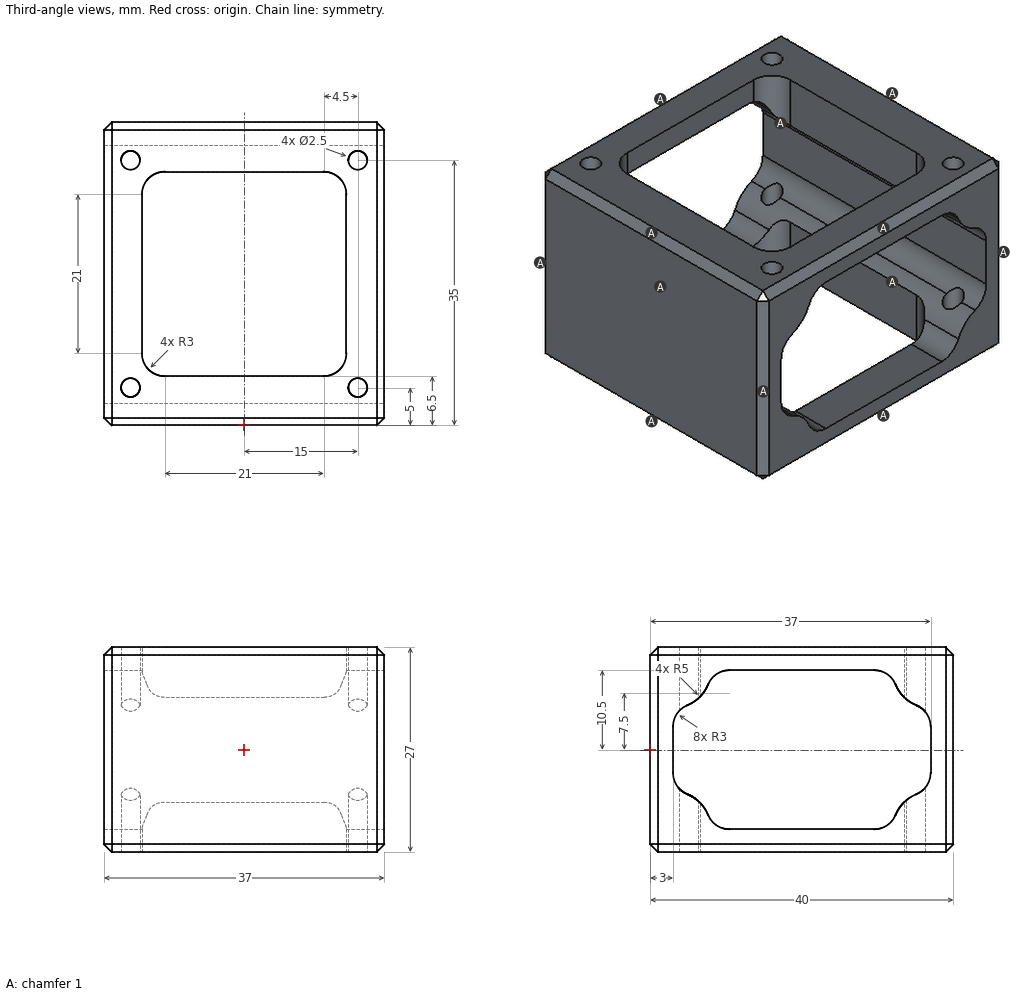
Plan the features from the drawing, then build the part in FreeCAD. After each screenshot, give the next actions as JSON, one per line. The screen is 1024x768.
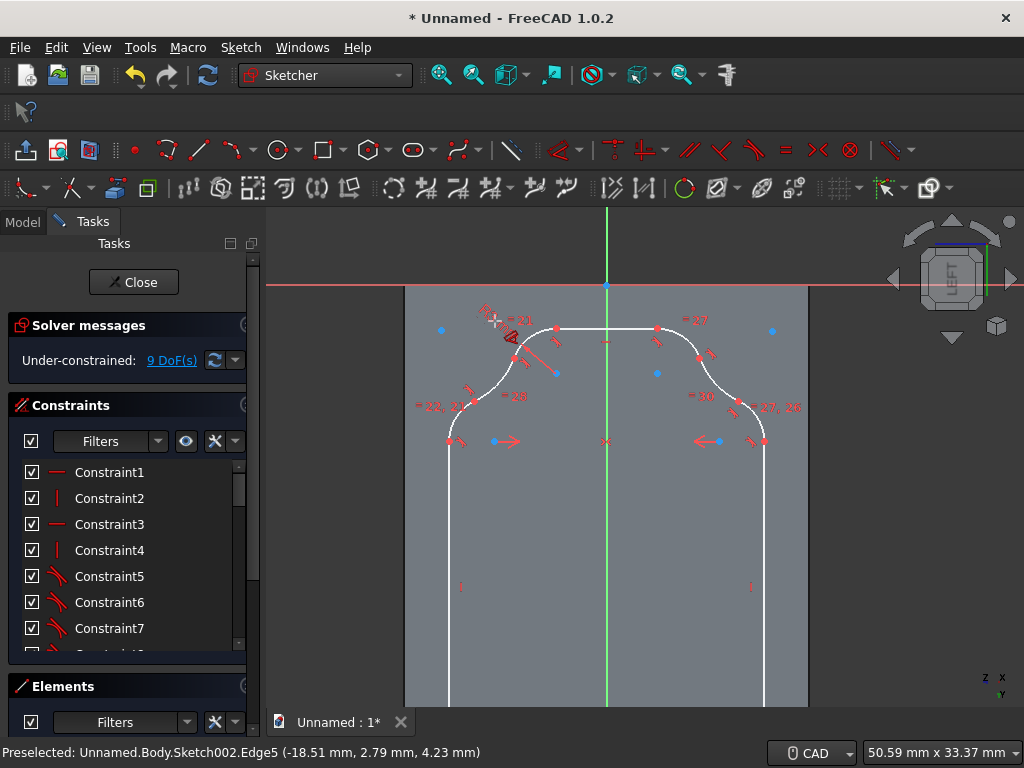
{"action": "left_click", "coordinate": [490, 392]}
{"action": "left_click", "coordinate": [510, 417]}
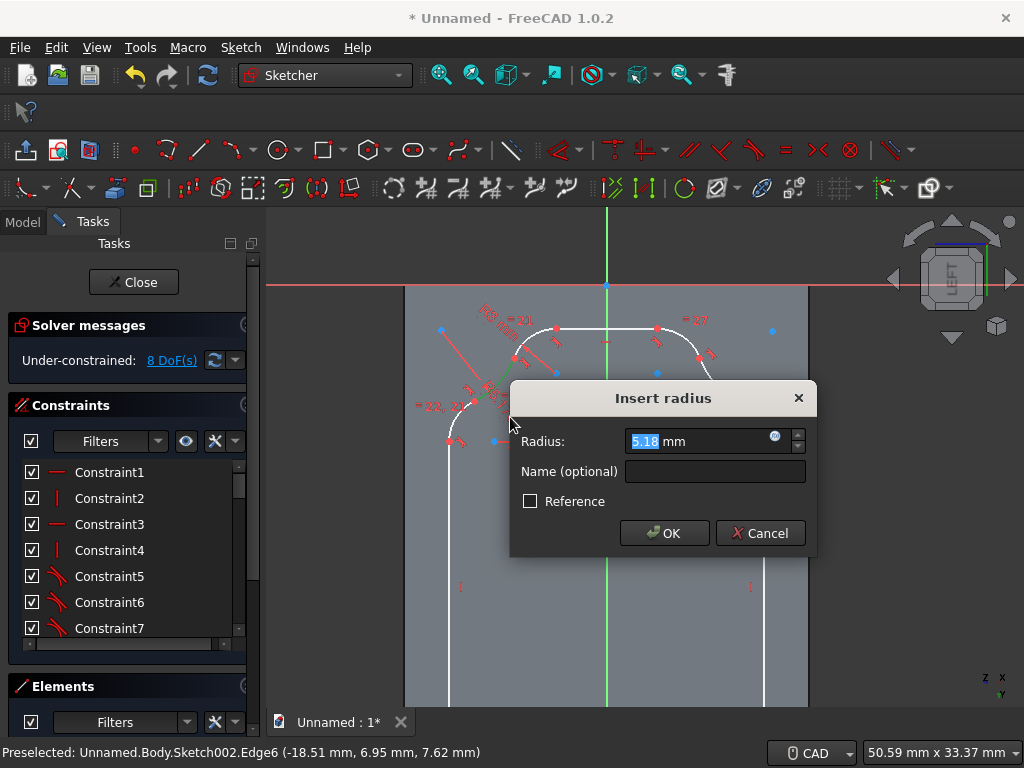
{"action": "type", "text": "5"}
{"action": "key", "text": "Return"}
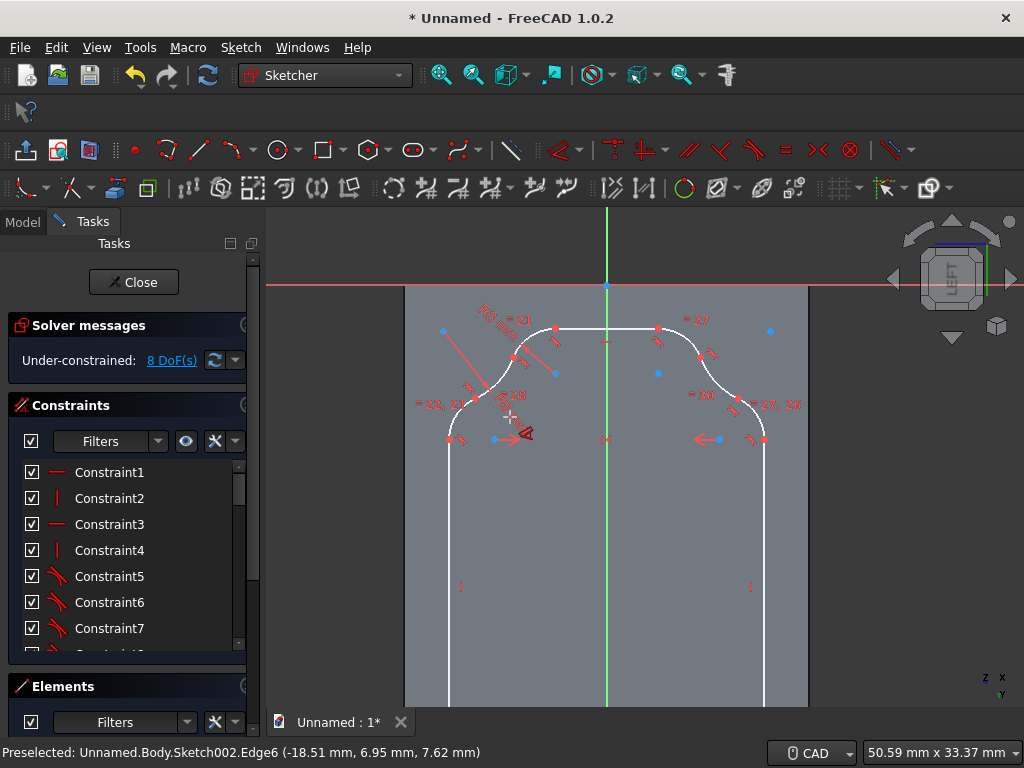
{"action": "left_click", "coordinate": [659, 329]}
{"action": "left_click", "coordinate": [693, 307]}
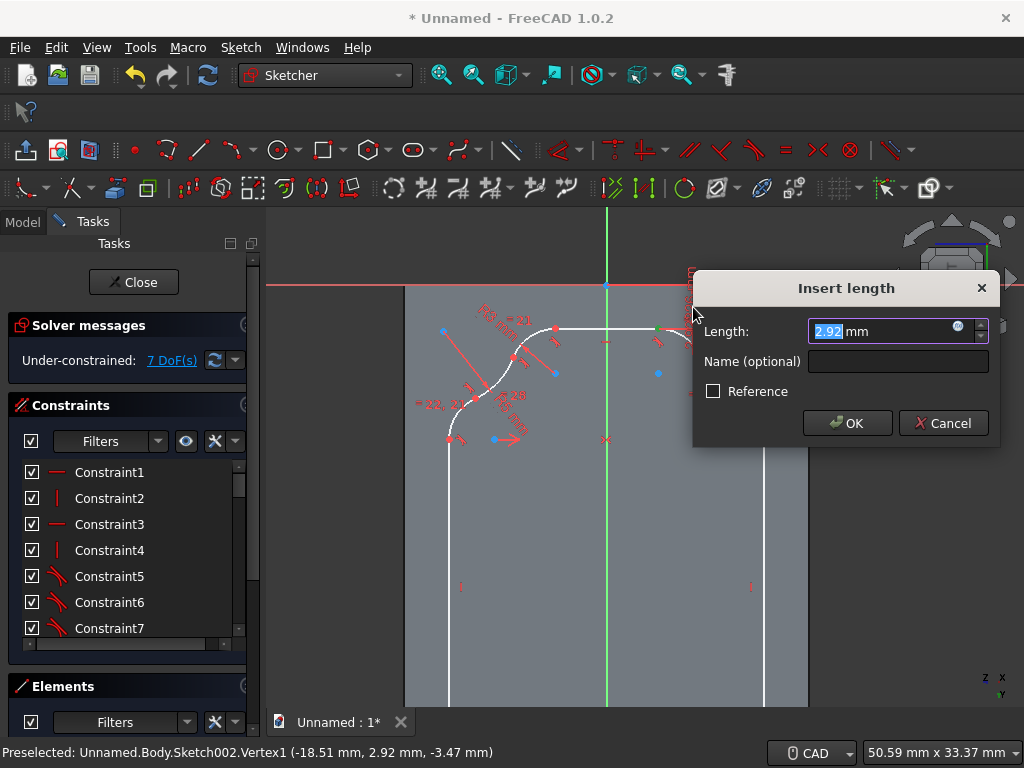
{"action": "type", "text": "3"}
{"action": "key", "text": "Return"}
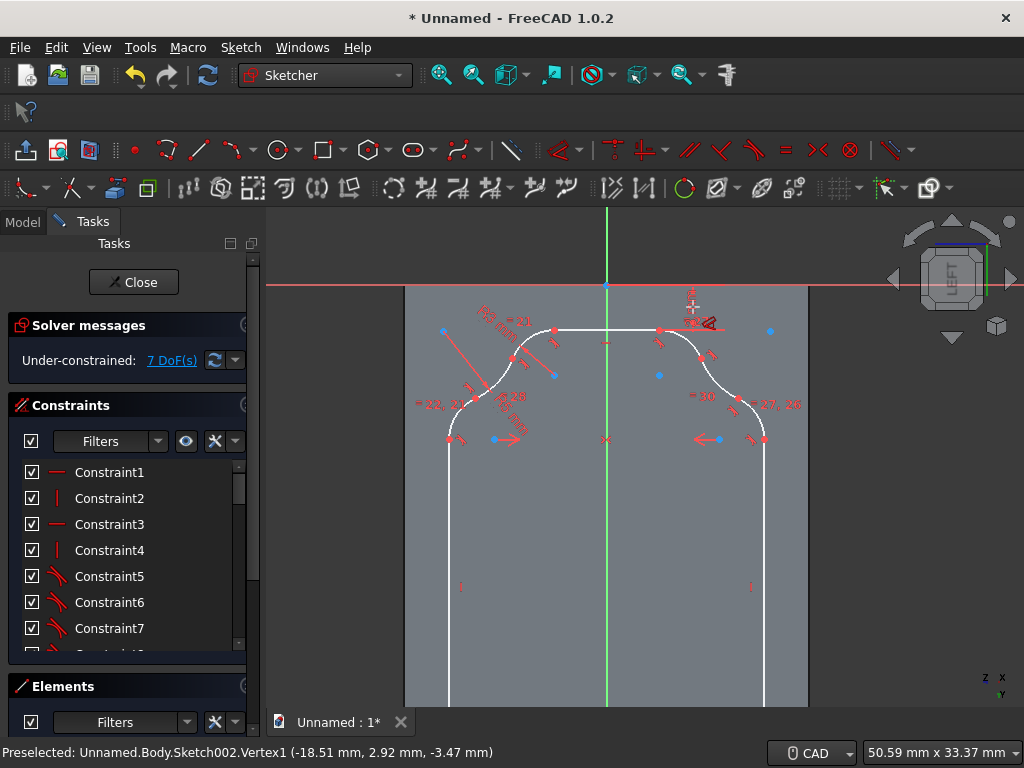
{"action": "left_click", "coordinate": [443, 331]}
{"action": "left_click", "coordinate": [409, 308]}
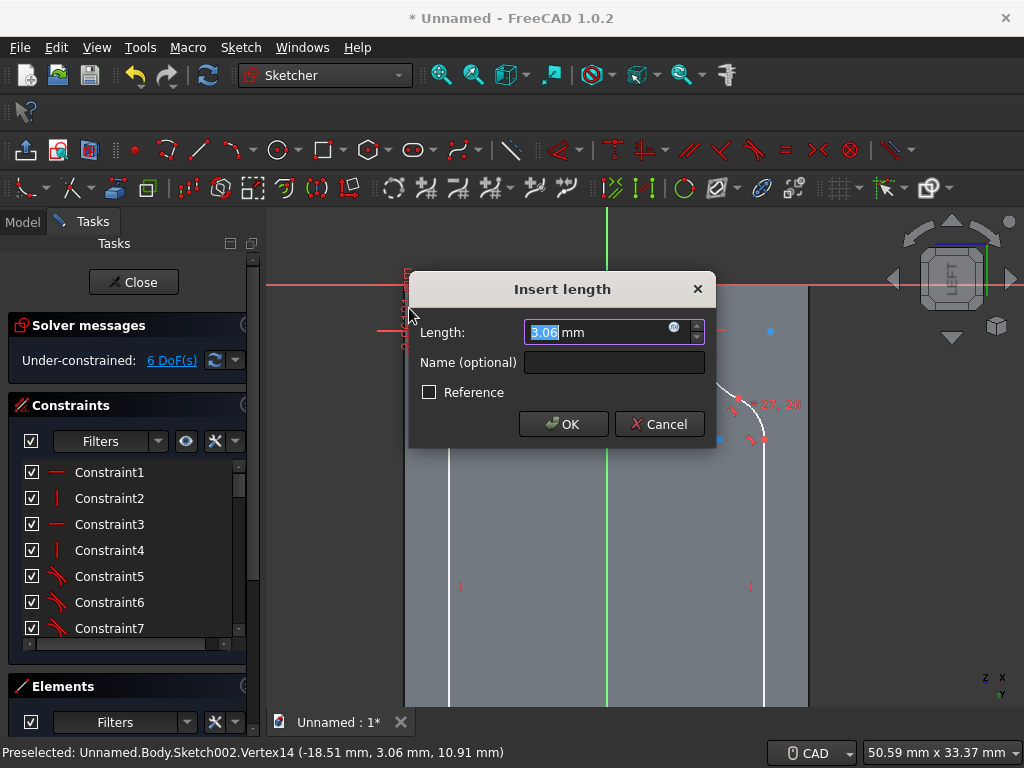
{"action": "type", "text": "3"}
{"action": "key", "text": "Return"}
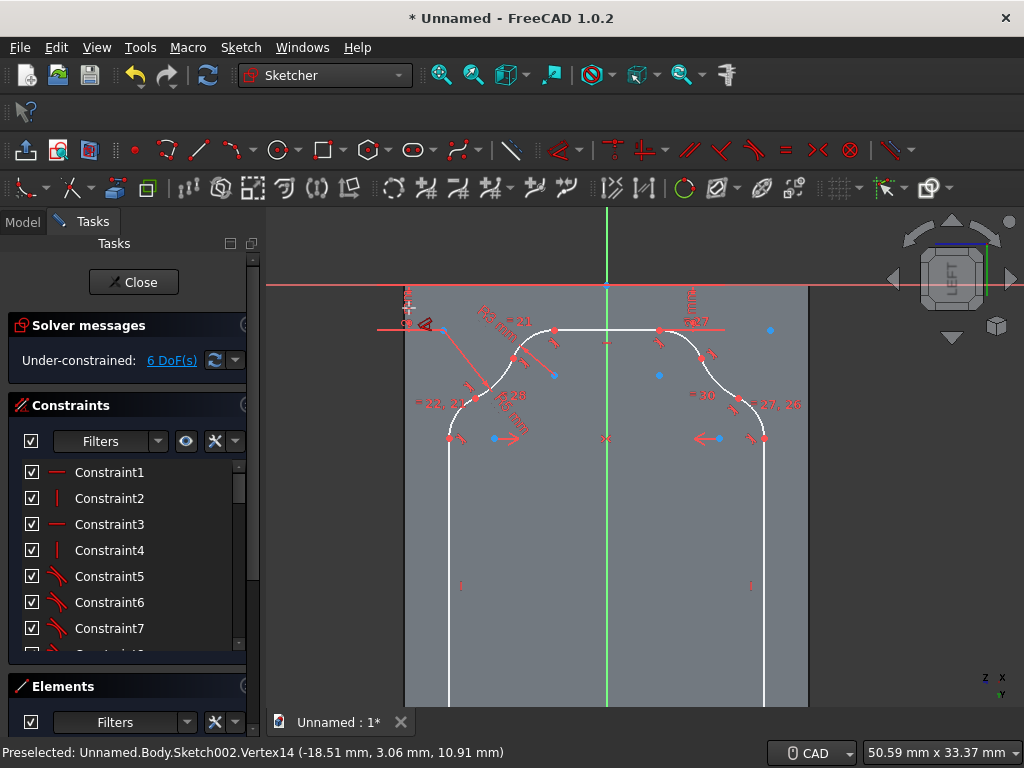
{"action": "left_click", "coordinate": [771, 331]}
{"action": "left_click", "coordinate": [805, 308]}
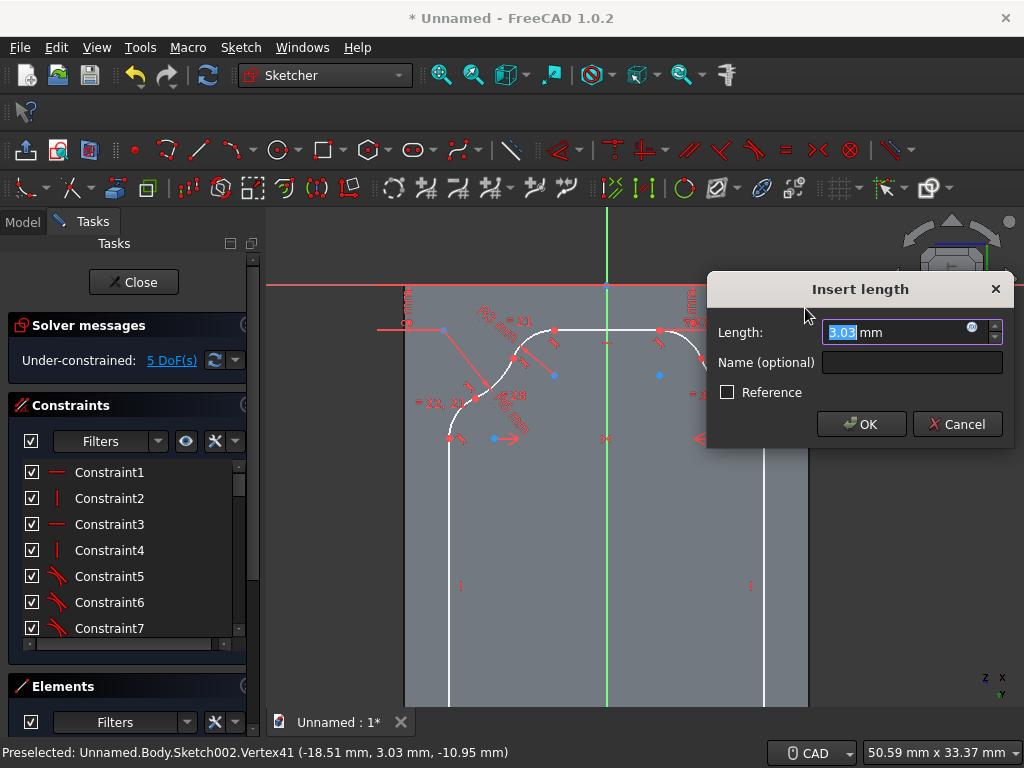
{"action": "type", "text": "3"}
{"action": "key", "text": "Return"}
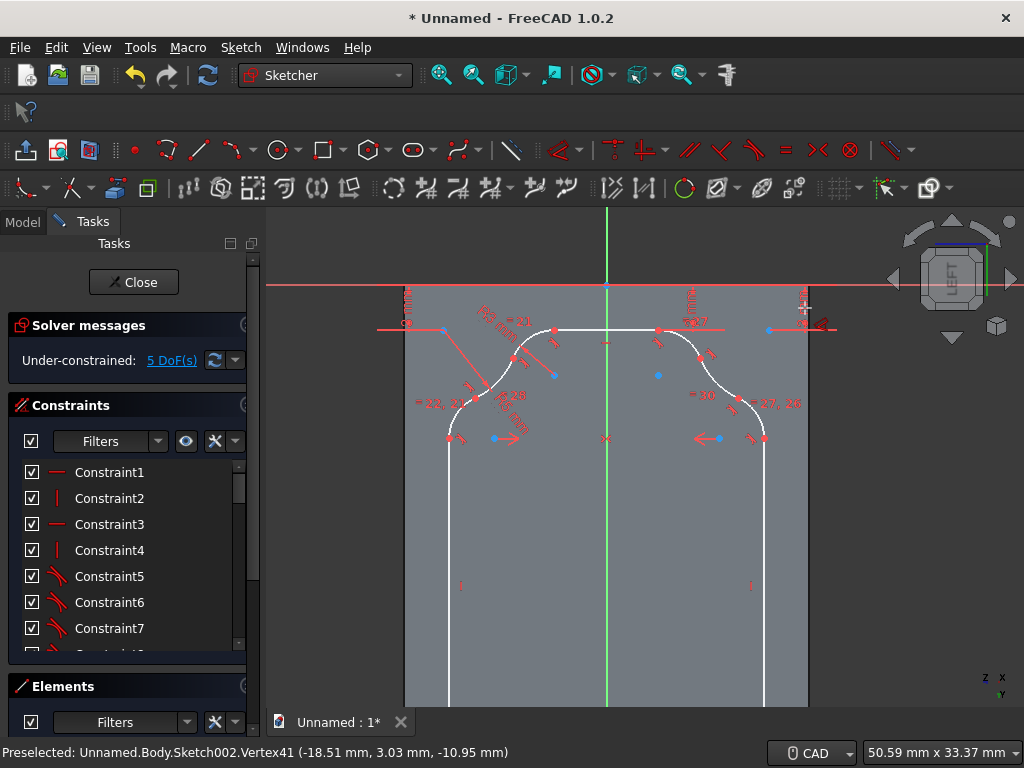
{"action": "scroll", "coordinate": [540, 329], "scroll_direction": "down", "scroll_amount": 3}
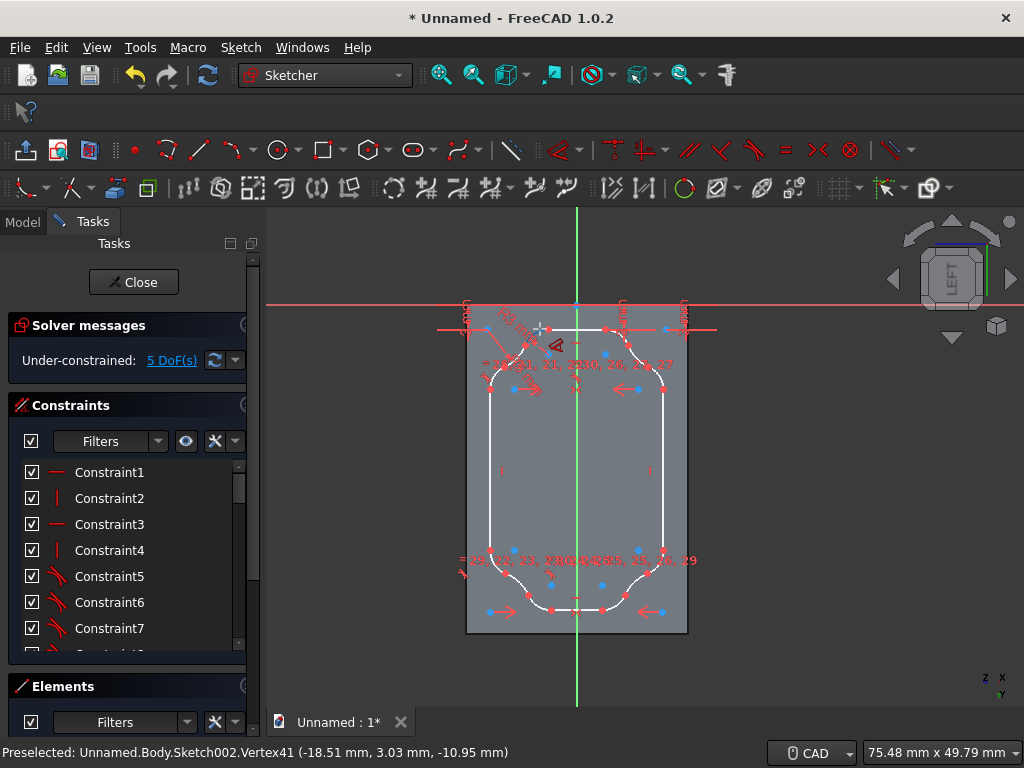
{"action": "left_click", "coordinate": [551, 610]}
{"action": "left_click", "coordinate": [517, 458]}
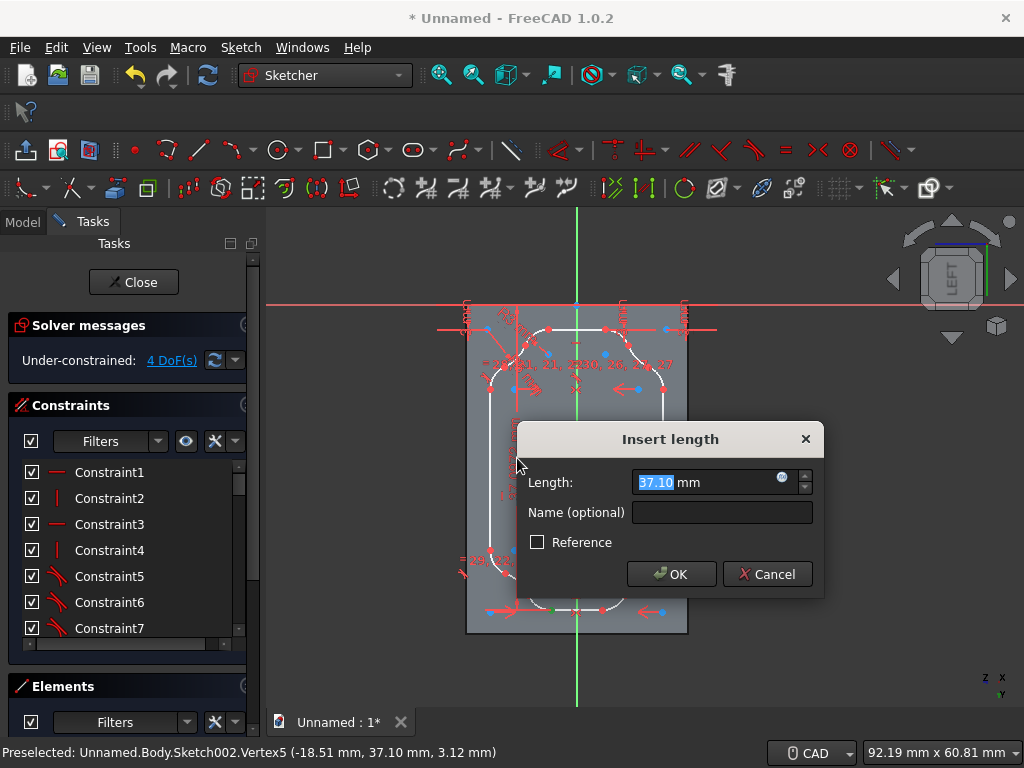
{"action": "type", "text": "37"}
{"action": "key", "text": "Return"}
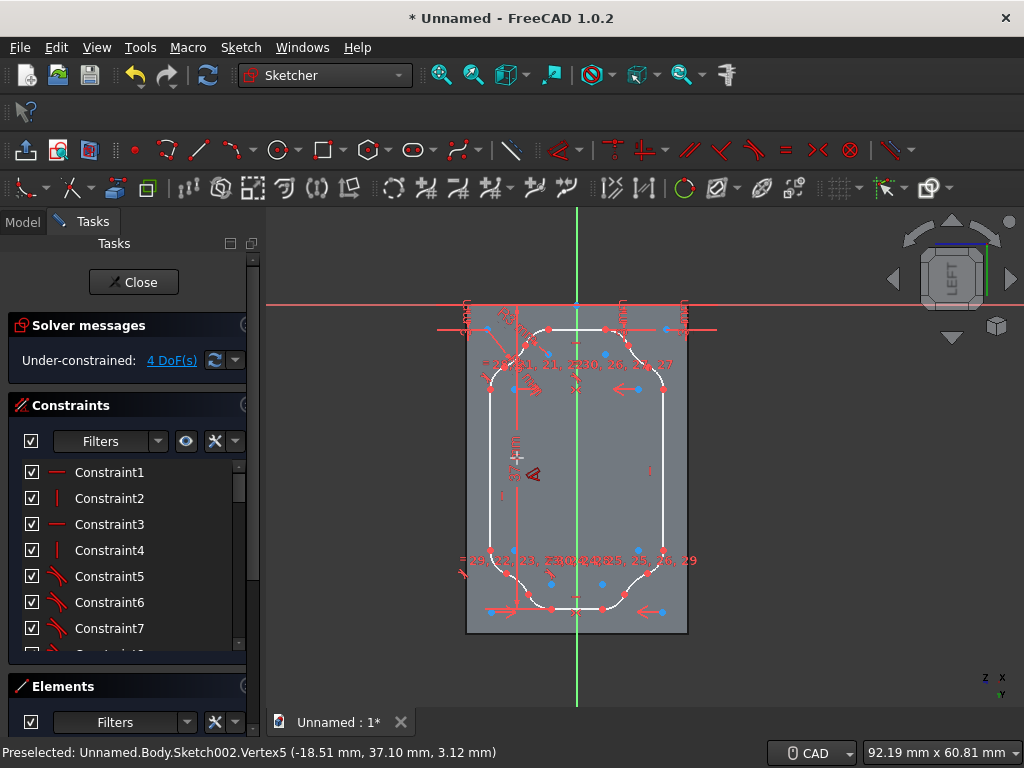
{"action": "left_click", "coordinate": [491, 612]}
{"action": "left_click", "coordinate": [457, 529]}